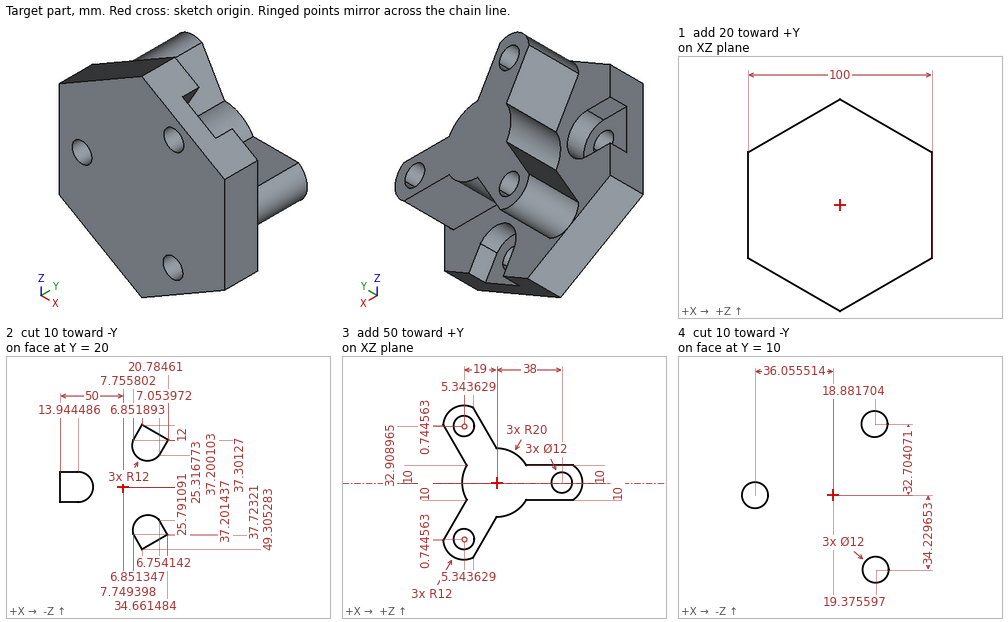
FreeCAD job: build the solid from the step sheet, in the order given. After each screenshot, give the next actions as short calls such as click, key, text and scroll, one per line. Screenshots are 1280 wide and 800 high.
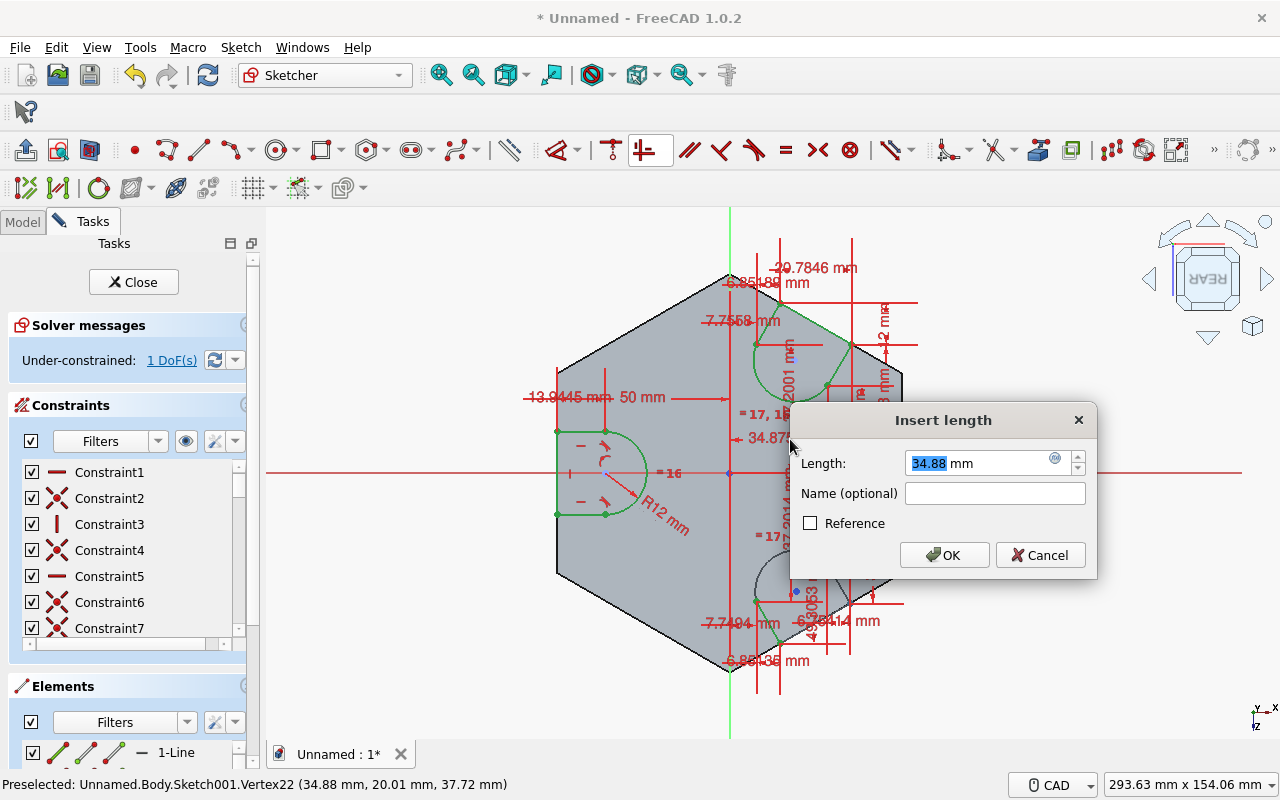
text(34.661484)
key(Return)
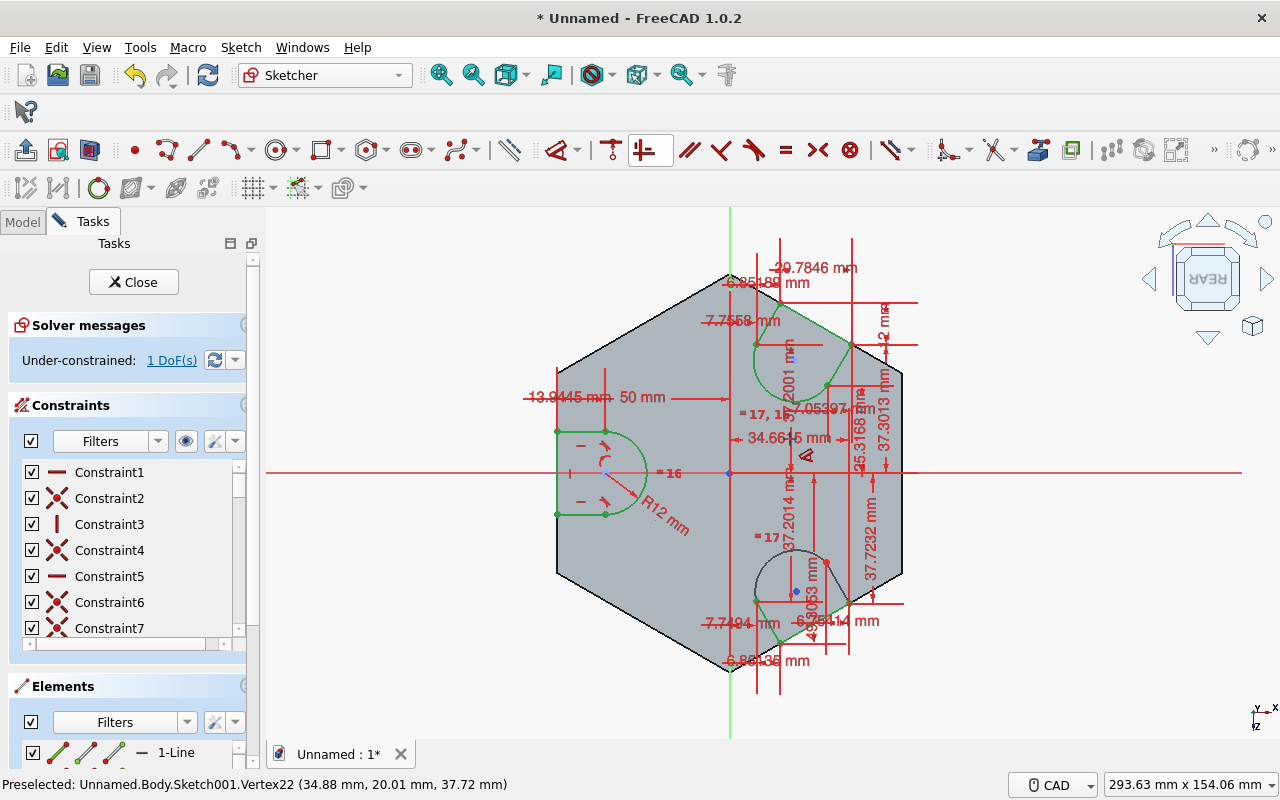
click(826, 563)
click(860, 487)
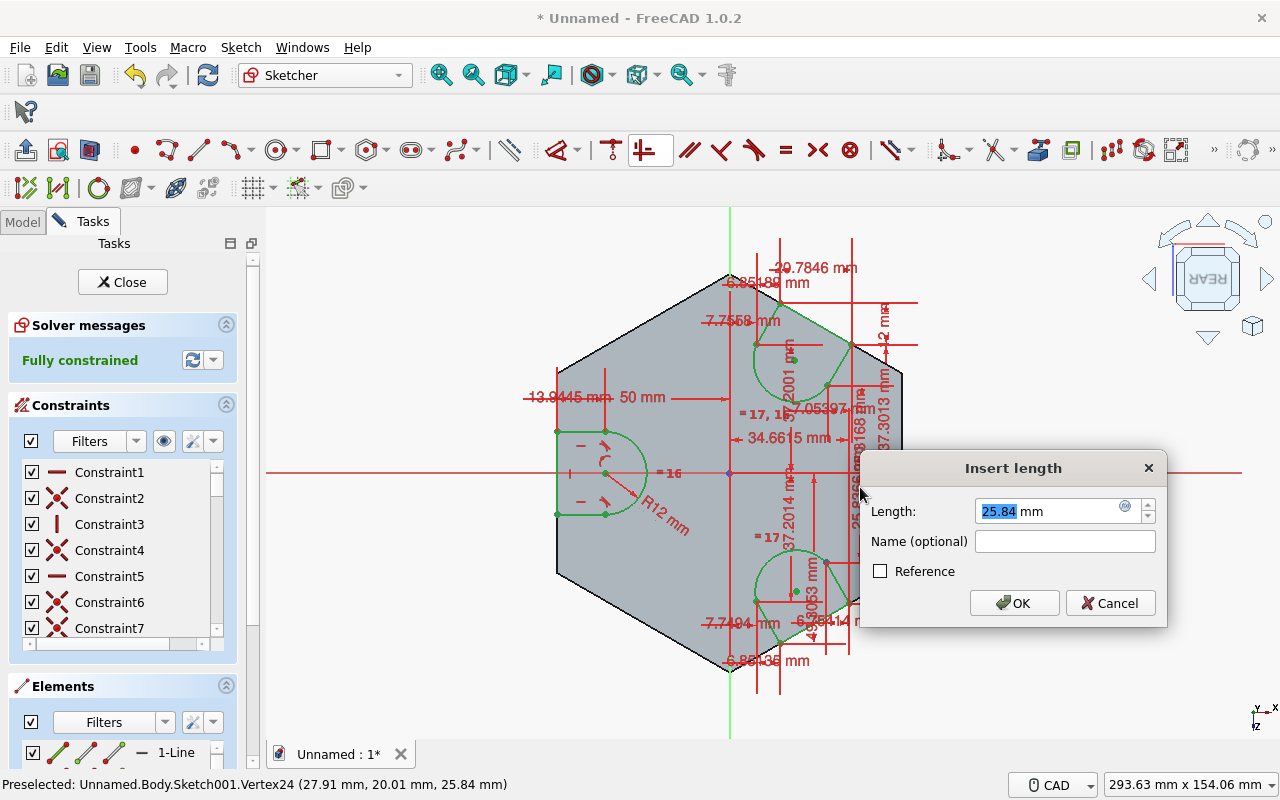
text(25.791091)
key(Return)
key(Escape)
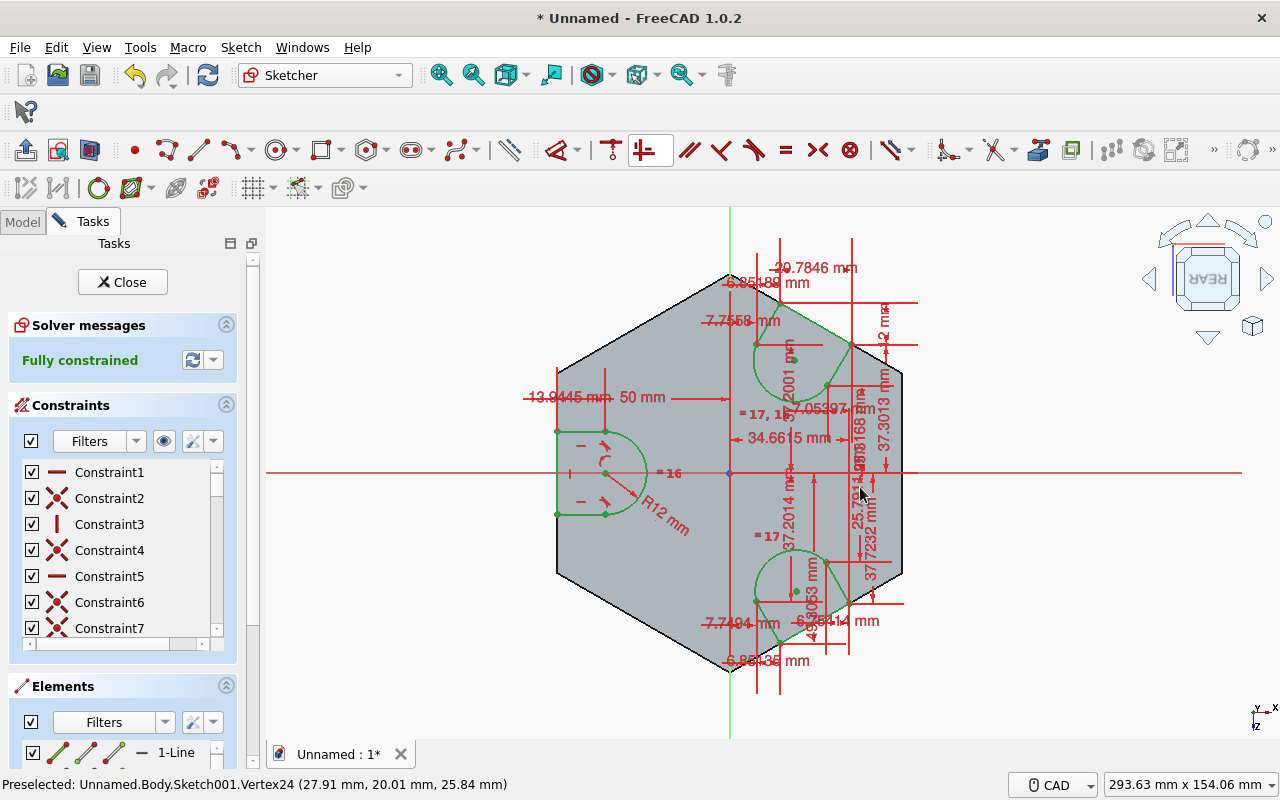
click(123, 282)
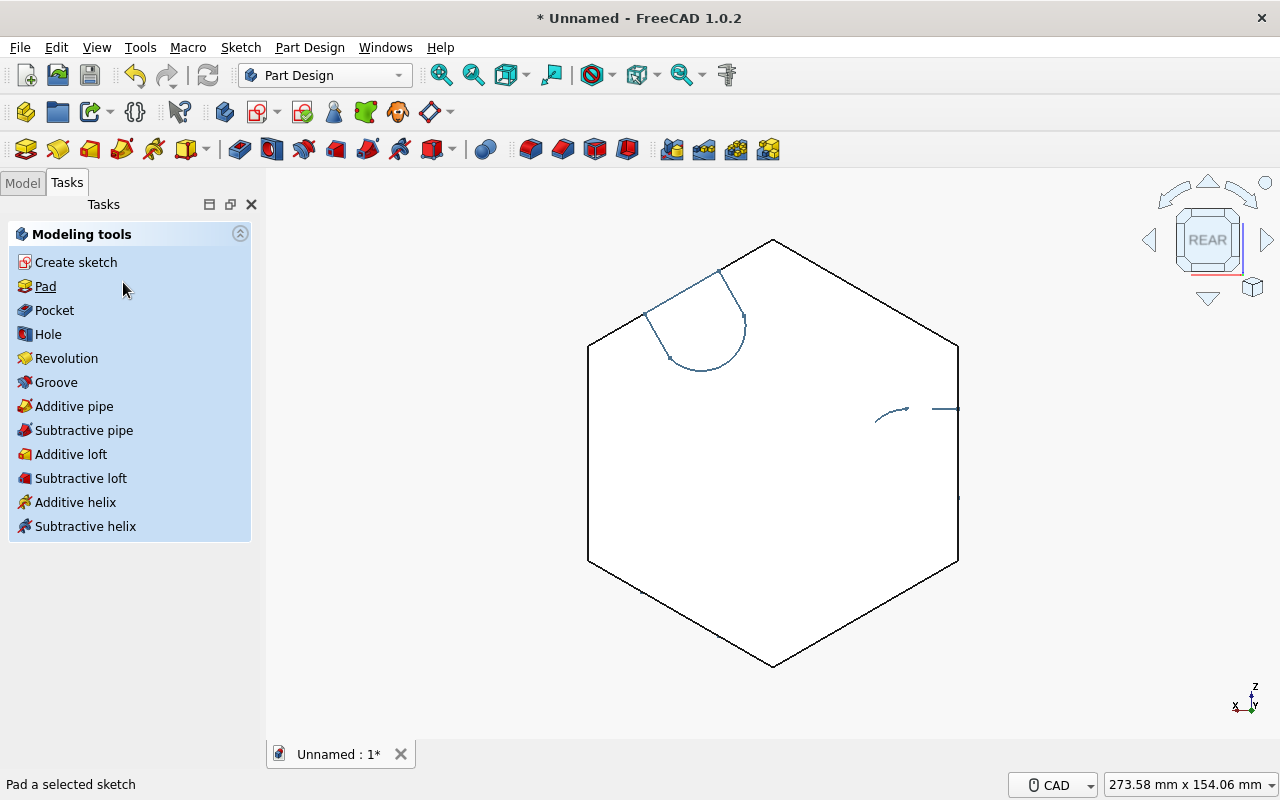
click(240, 150)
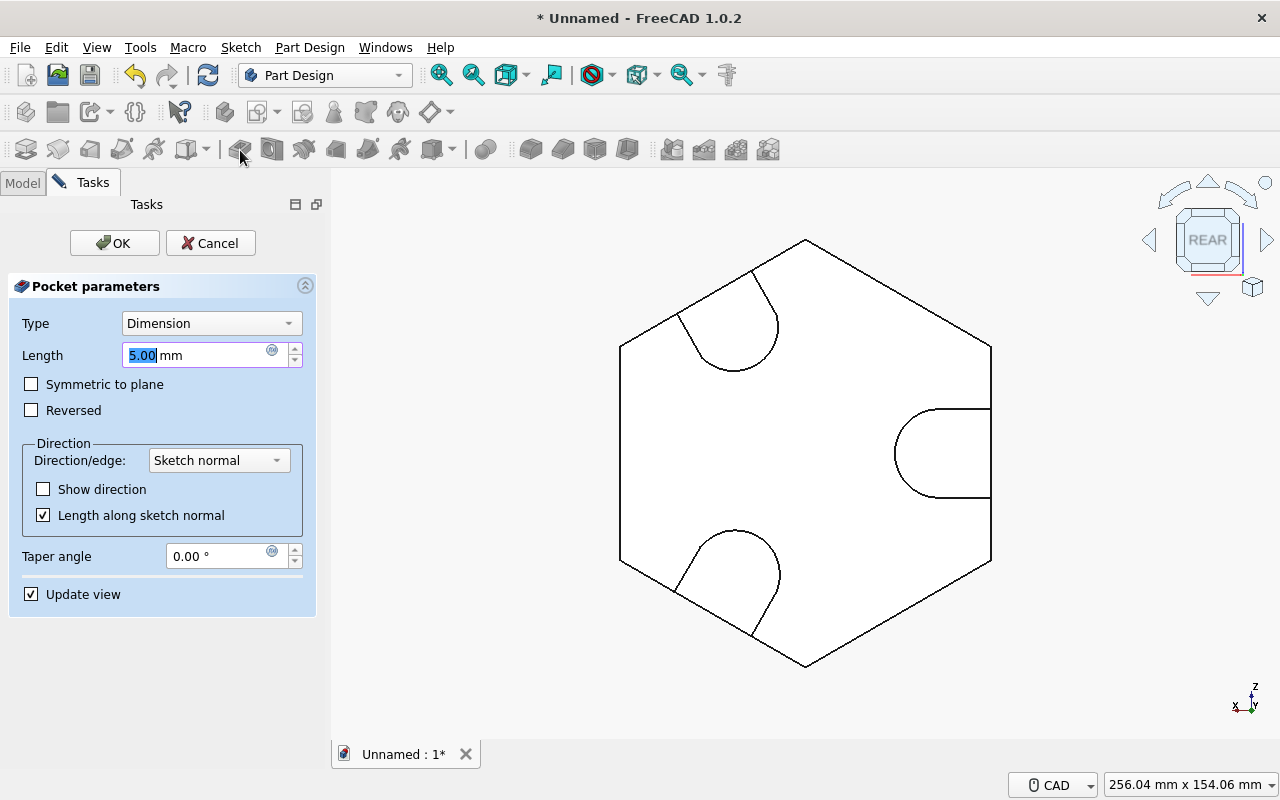
text(10)
key(Tab)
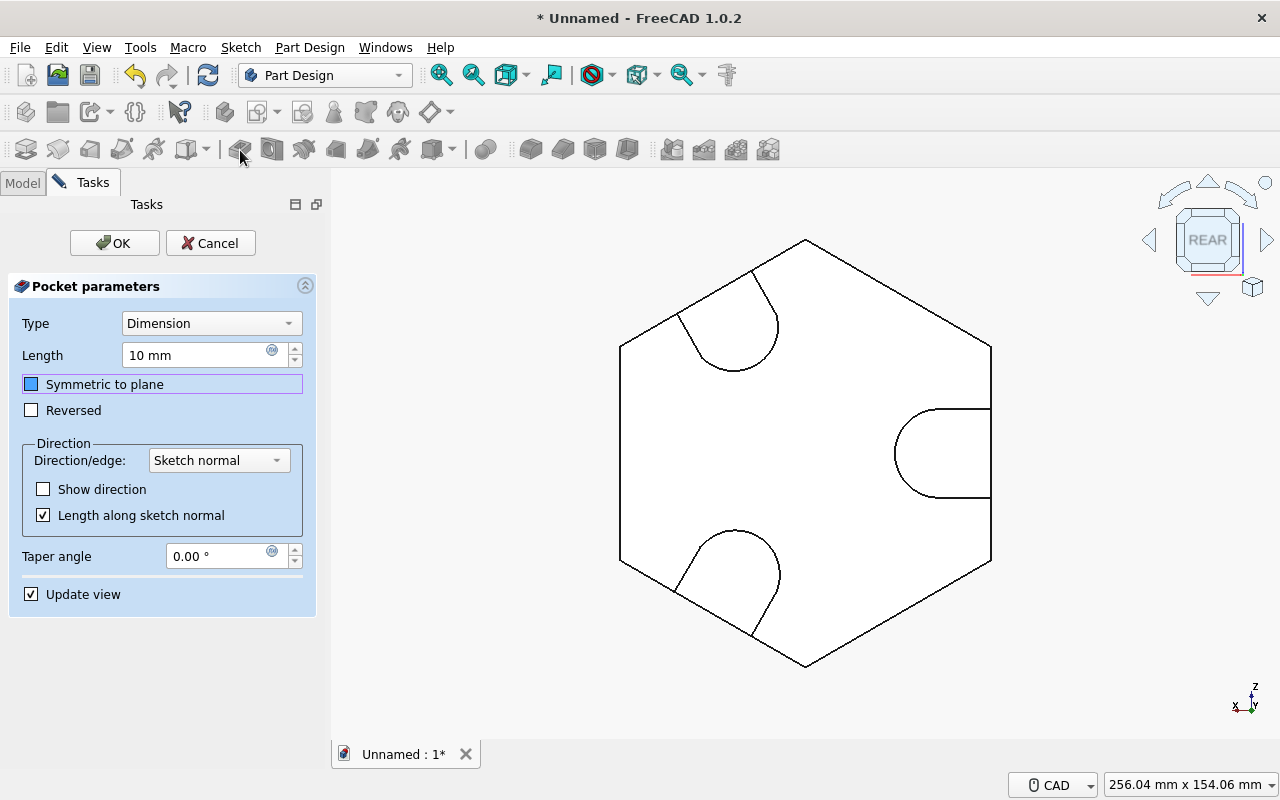
click(115, 243)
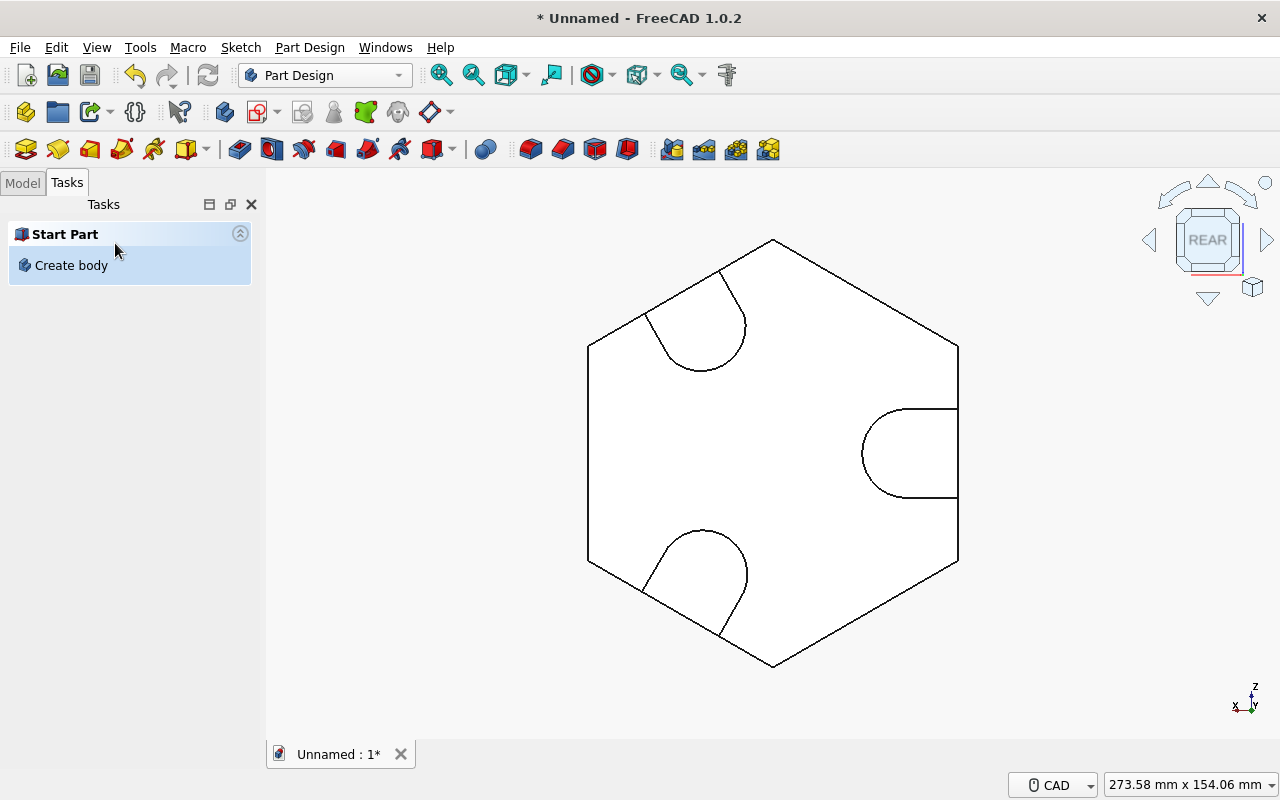
click(258, 112)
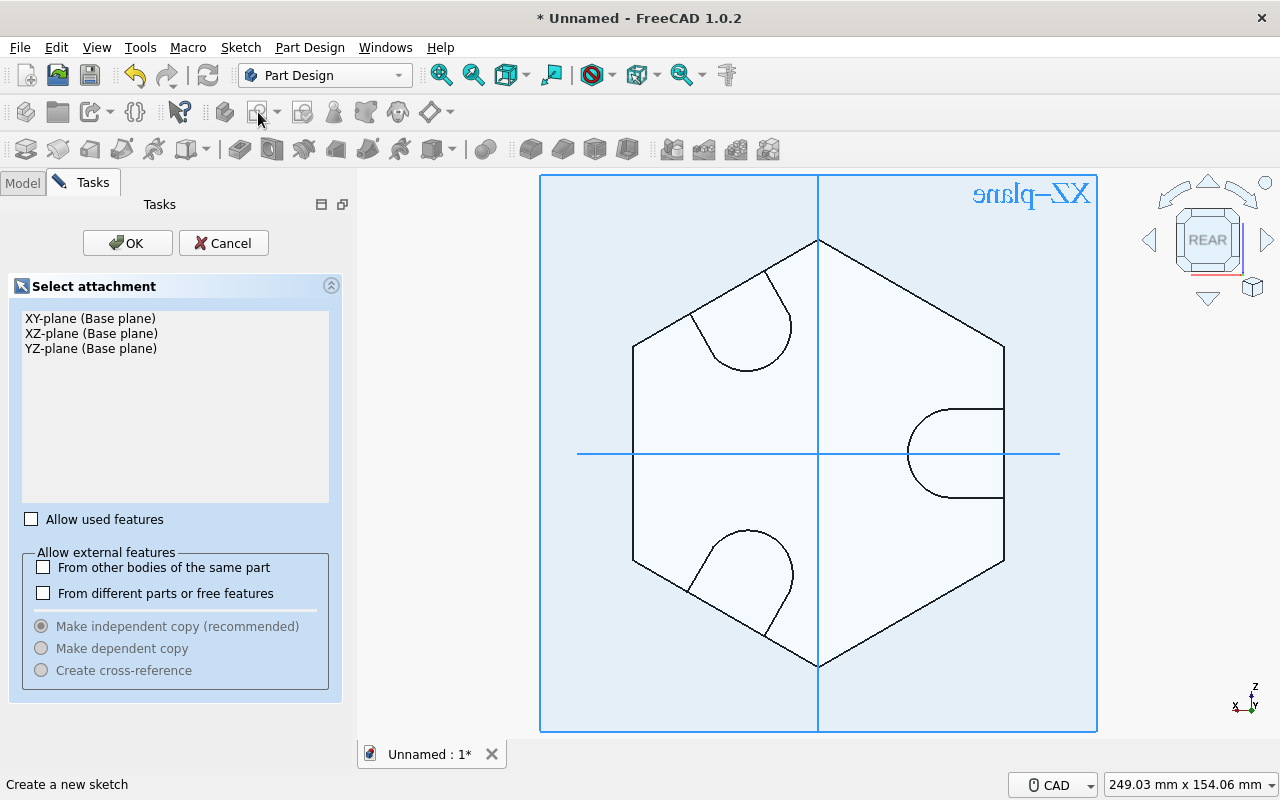
click(82, 334)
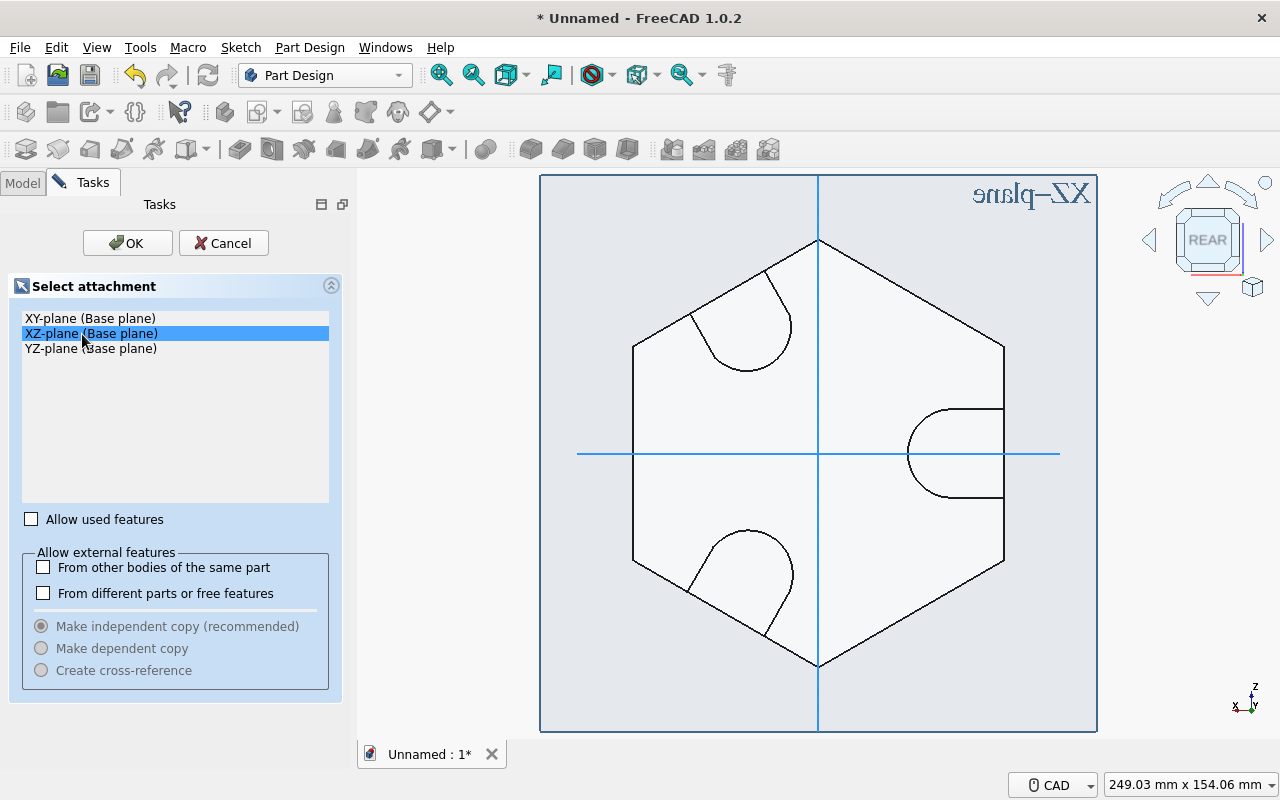
click(128, 243)